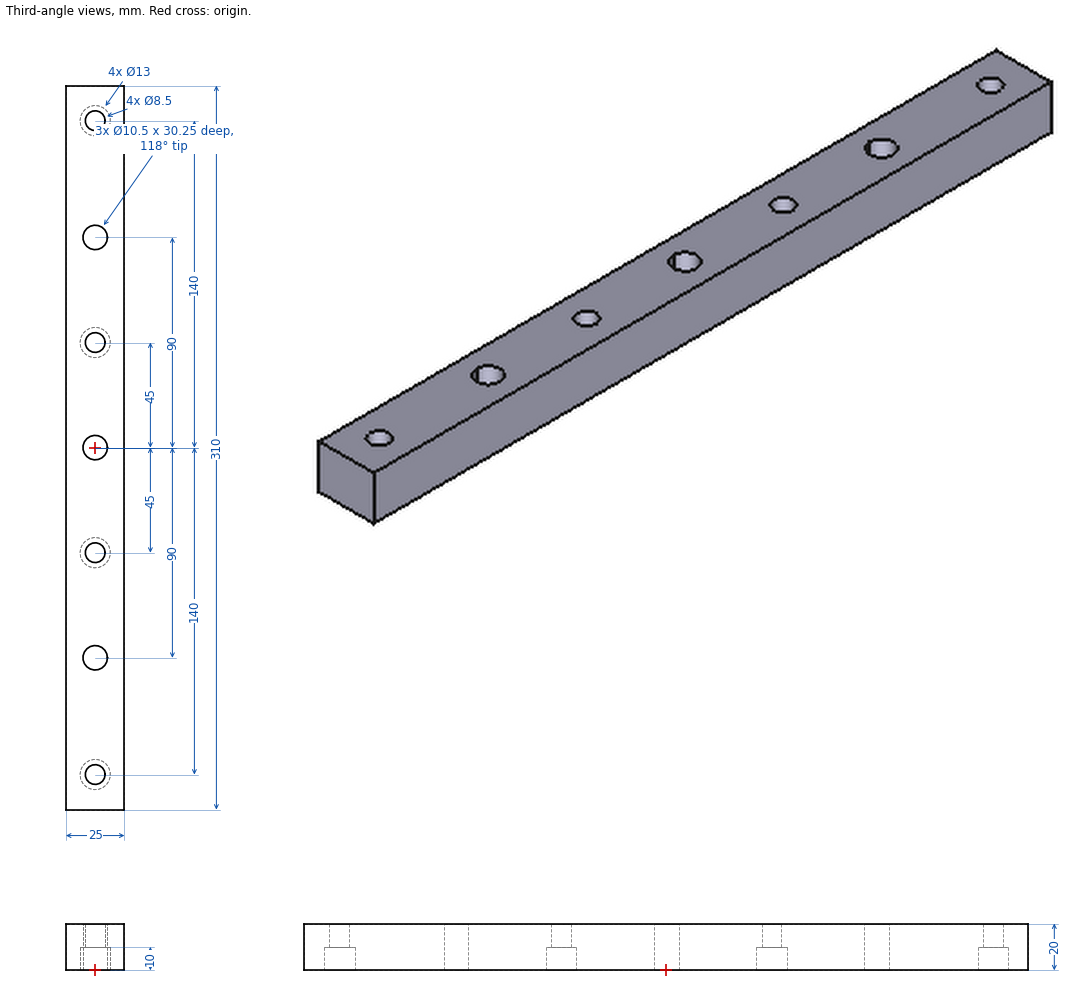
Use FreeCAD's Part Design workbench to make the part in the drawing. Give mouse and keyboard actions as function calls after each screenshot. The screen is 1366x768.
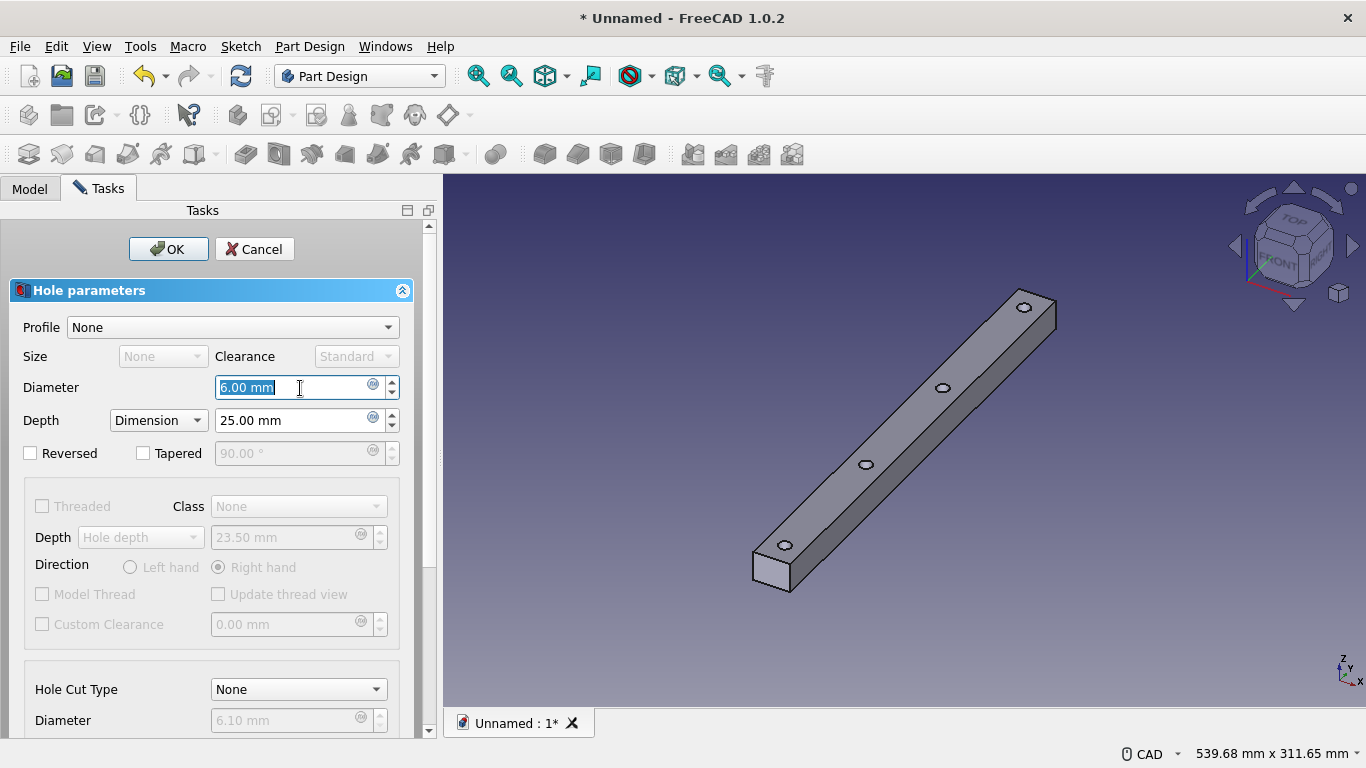
text(10.5)
key(Tab)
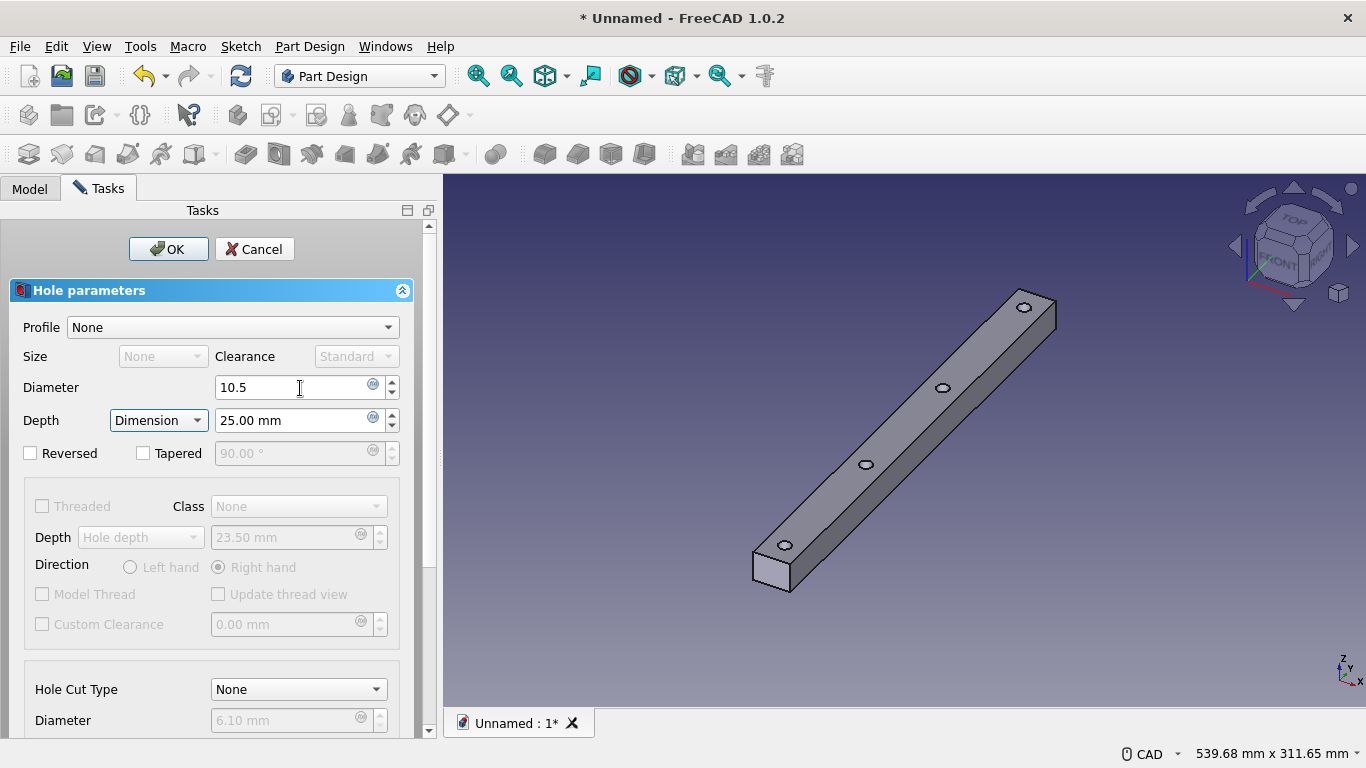
triple_click(300, 420)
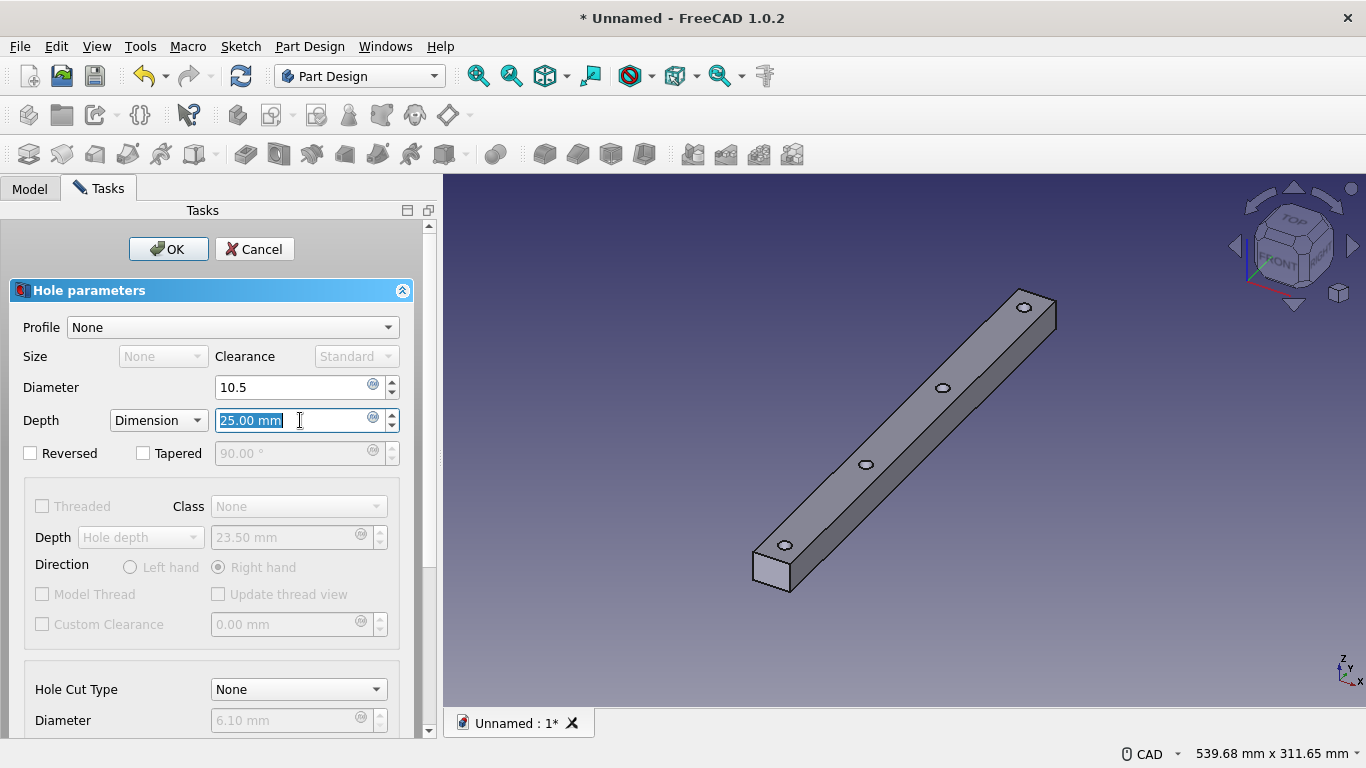
text(30.25)
key(Tab)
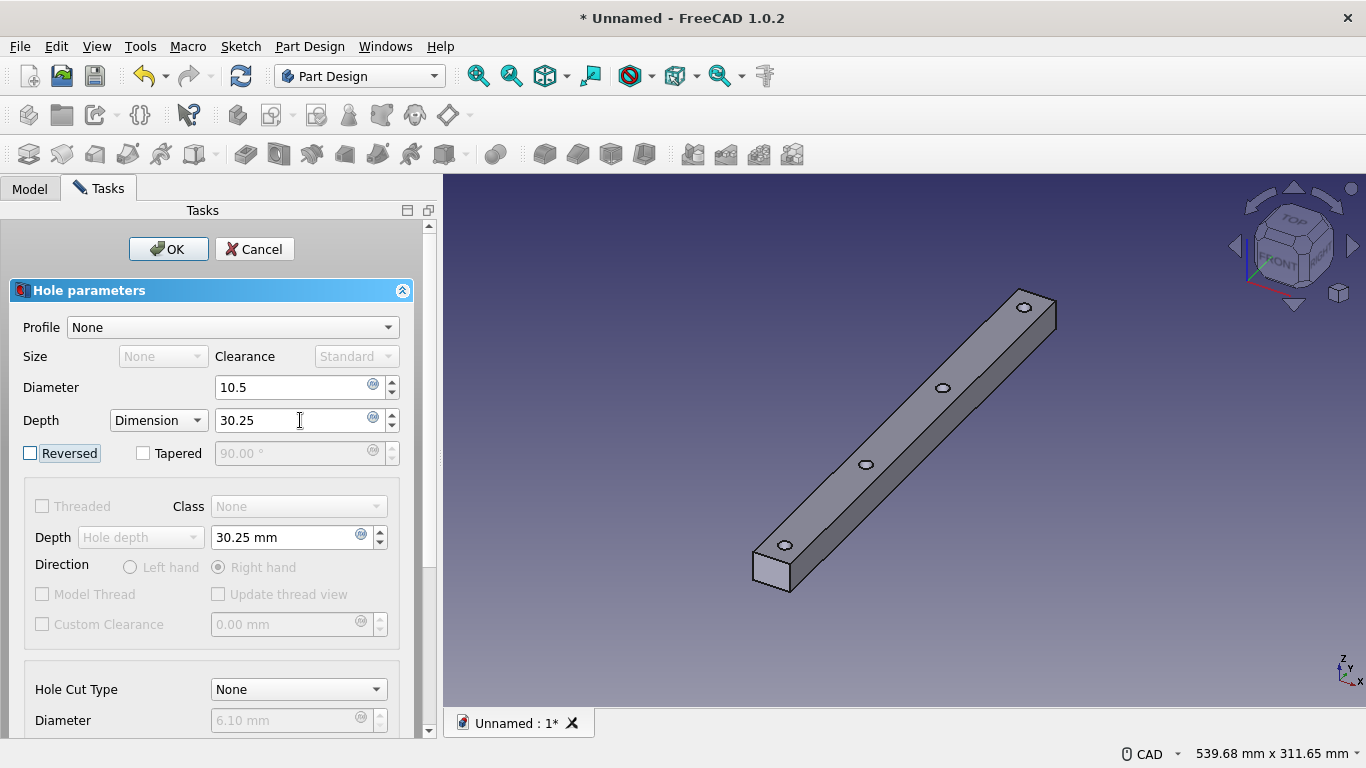
click(31, 453)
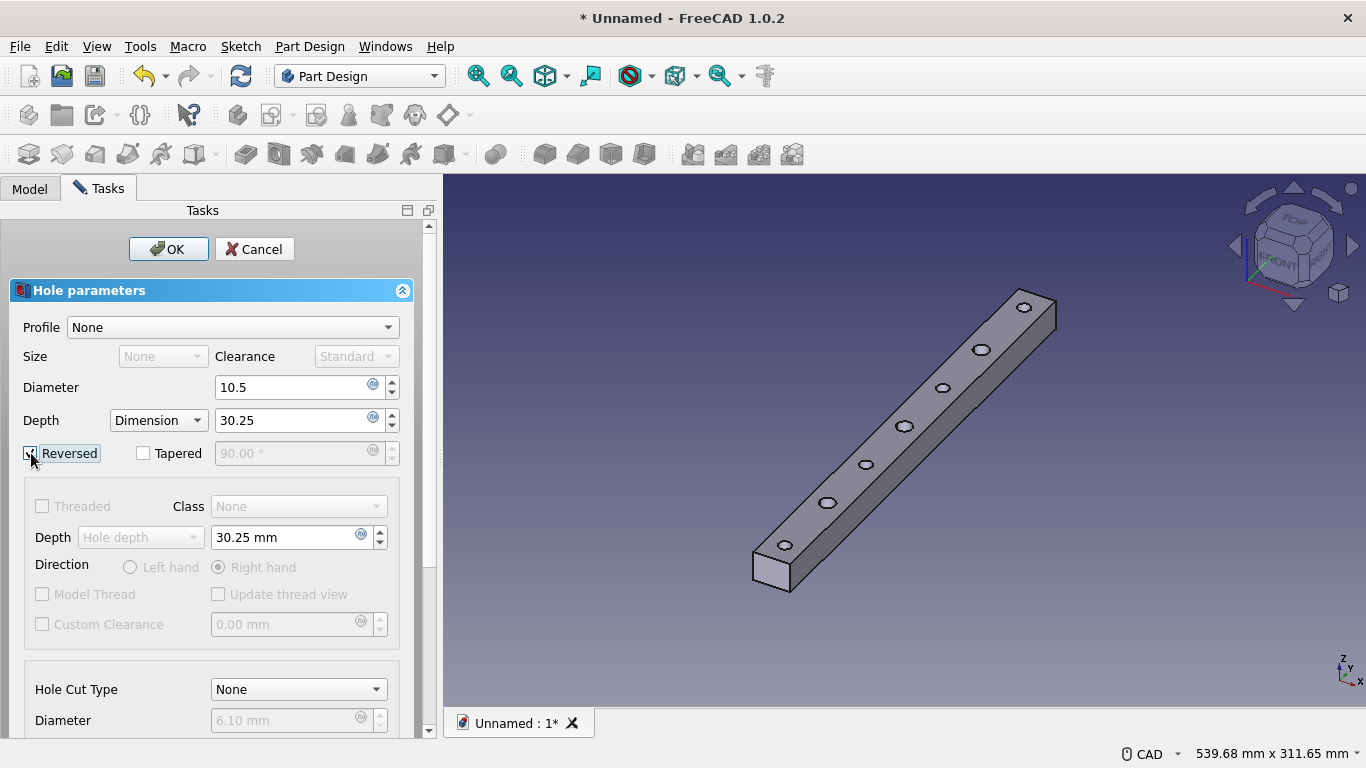
click(169, 249)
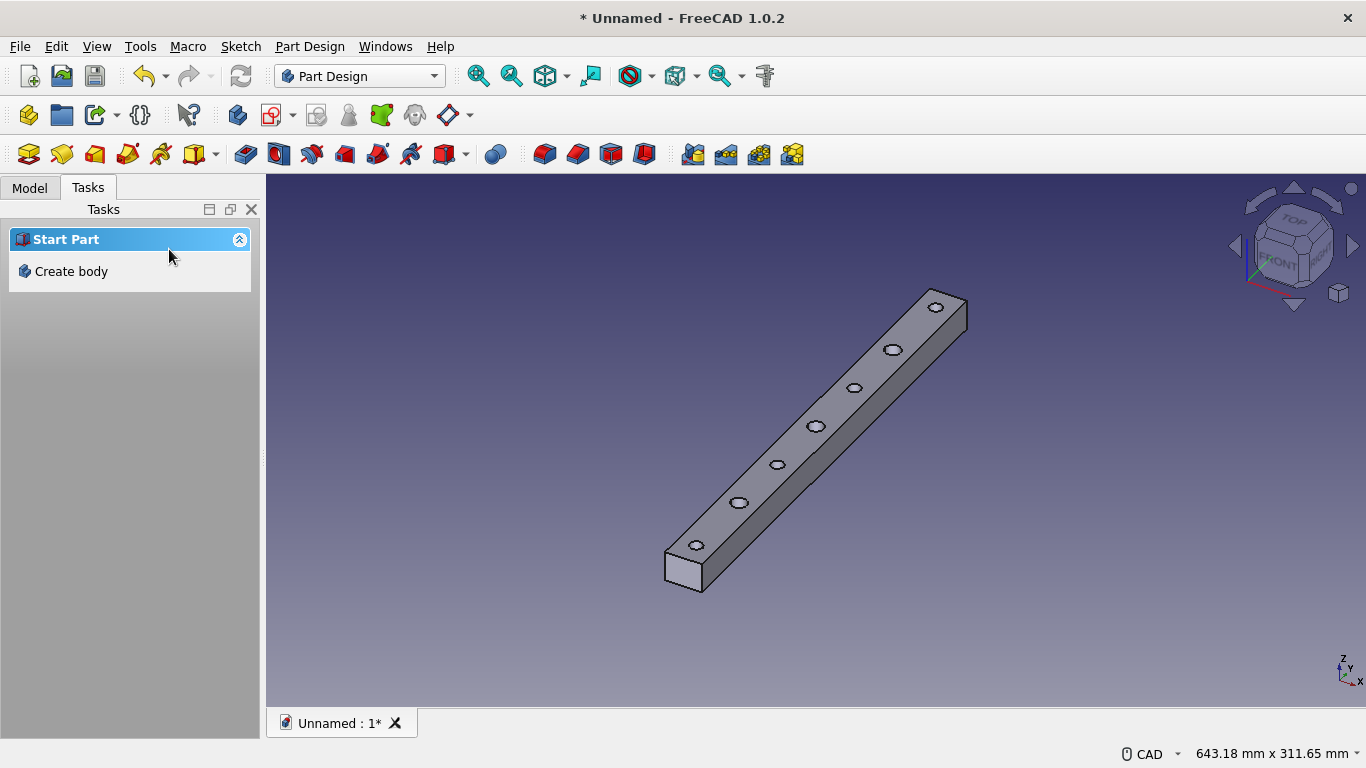
key(0)